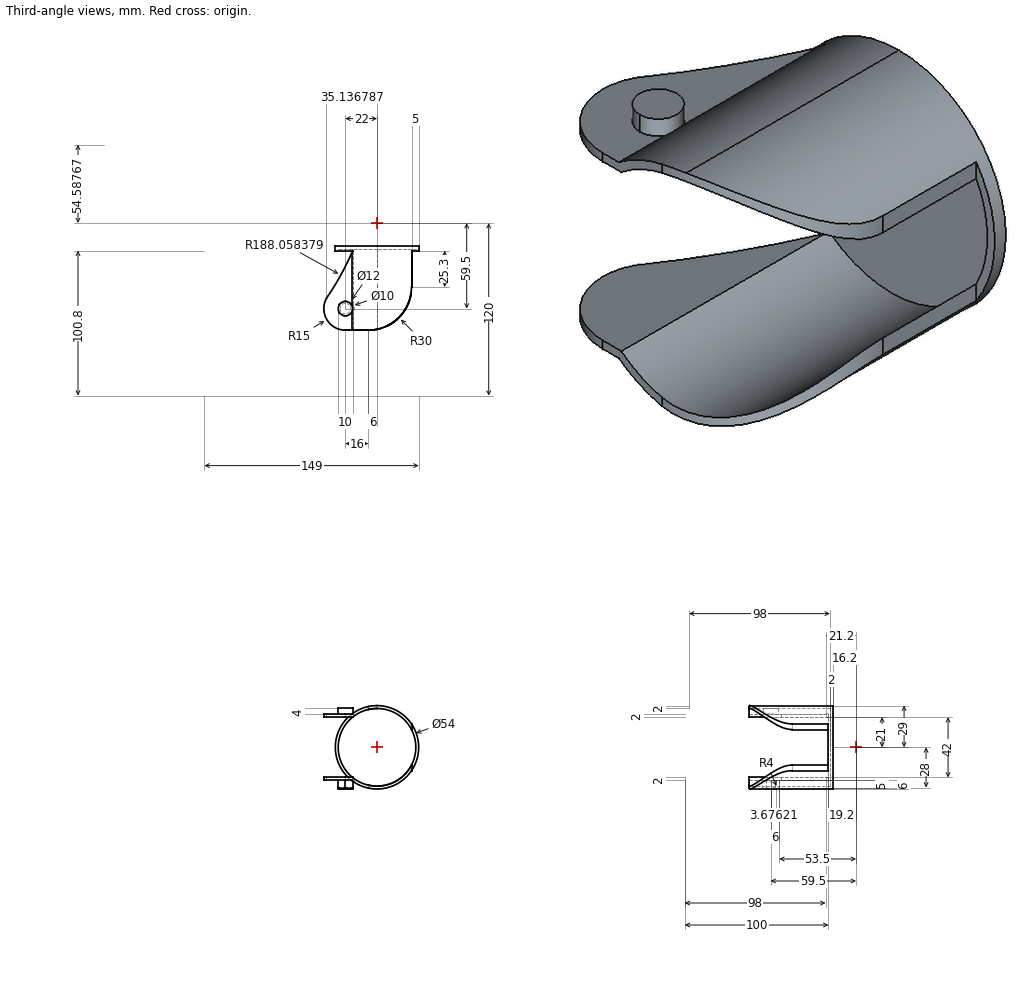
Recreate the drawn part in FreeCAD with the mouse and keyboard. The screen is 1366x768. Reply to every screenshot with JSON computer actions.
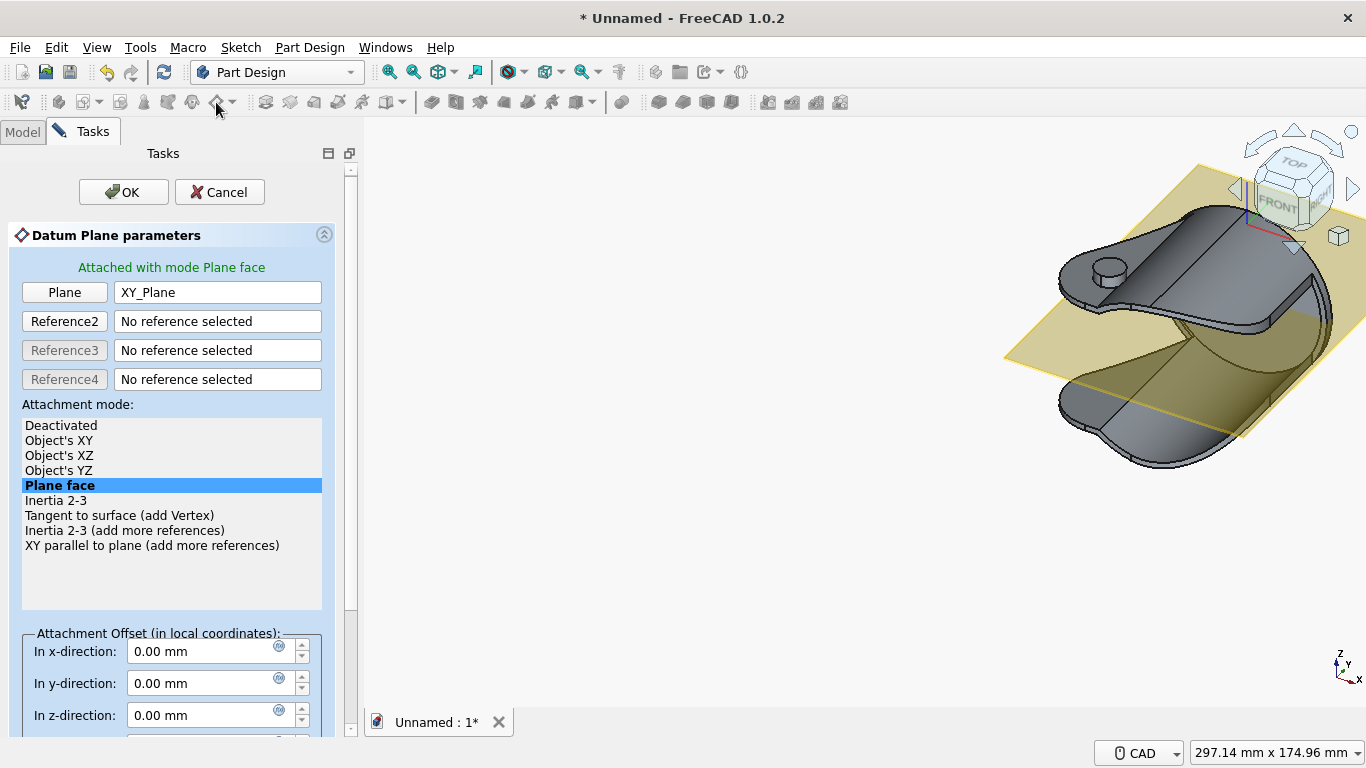
{"action": "triple_click", "coordinate": [210, 715]}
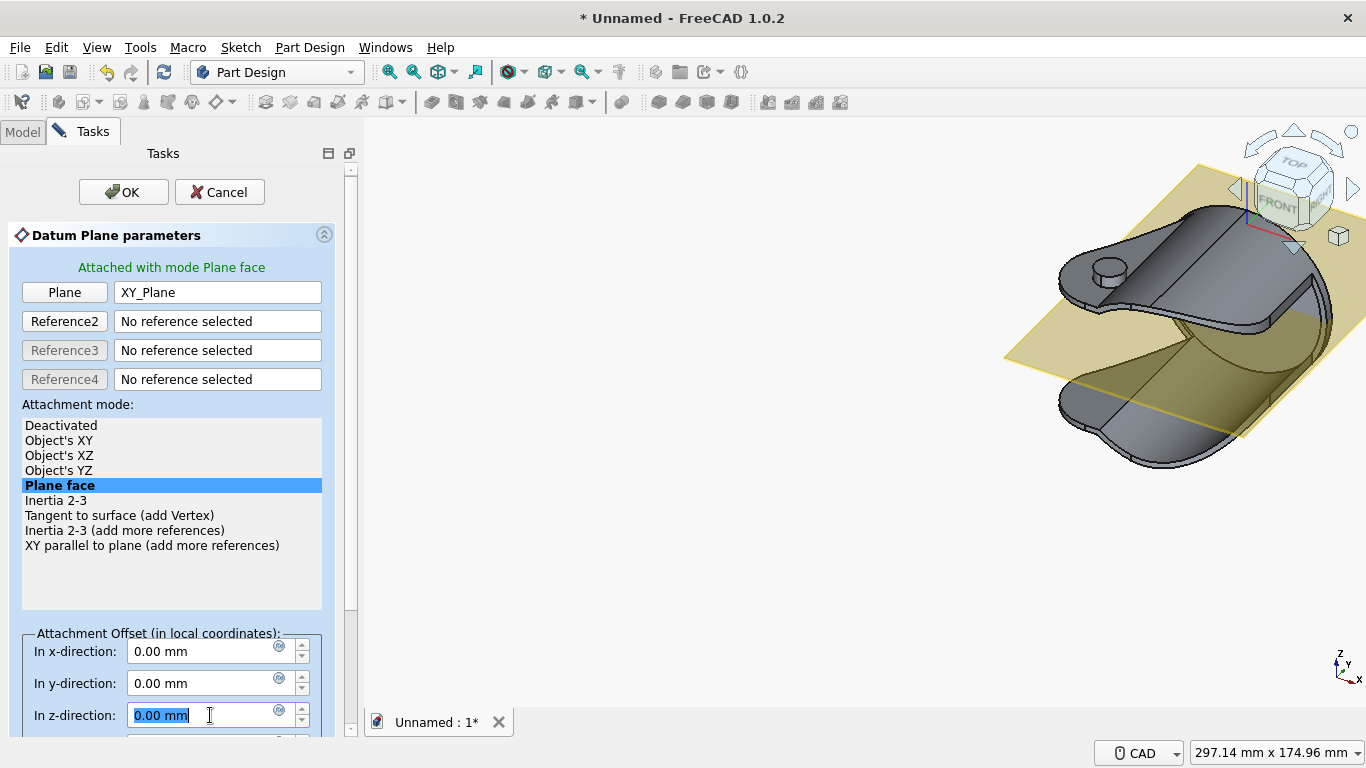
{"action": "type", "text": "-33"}
{"action": "key", "text": "Tab"}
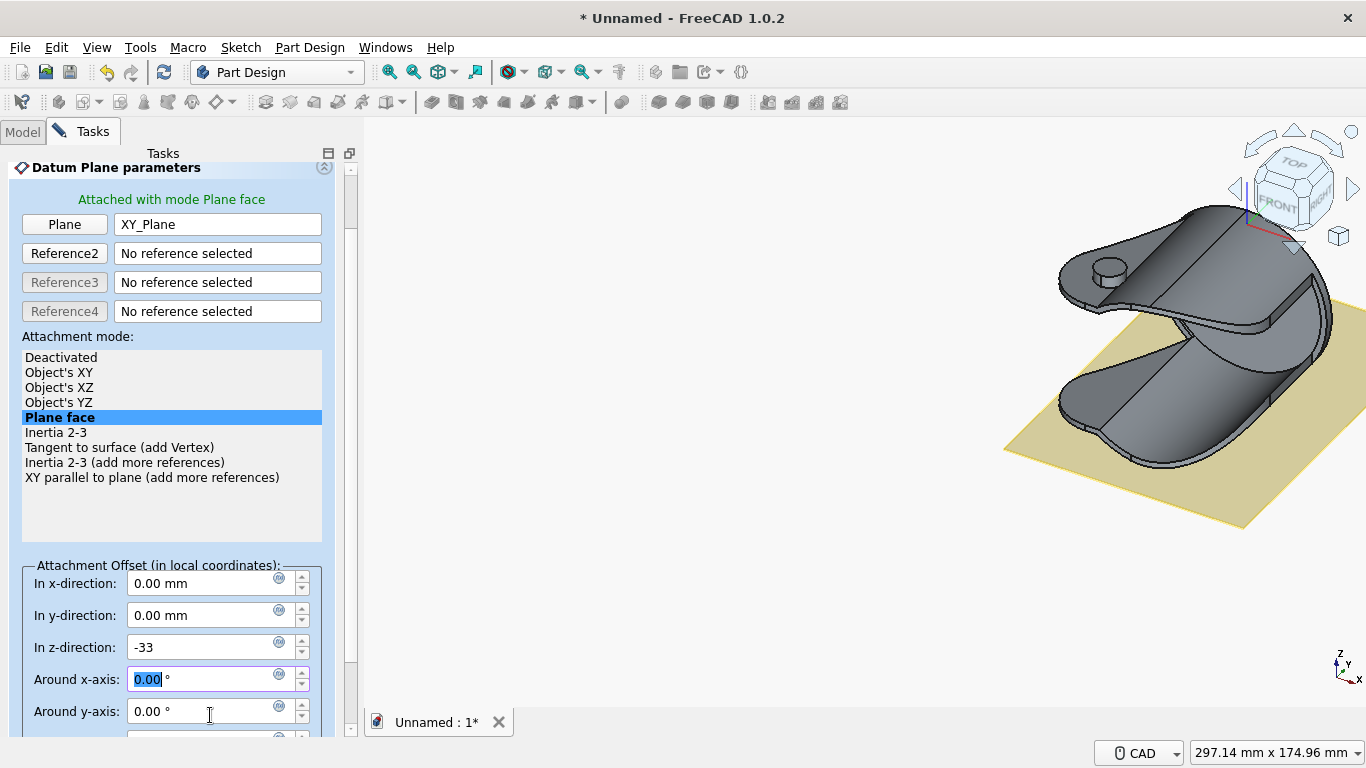
{"action": "scroll", "coordinate": [351, 450], "scroll_direction": "up", "scroll_amount": 2}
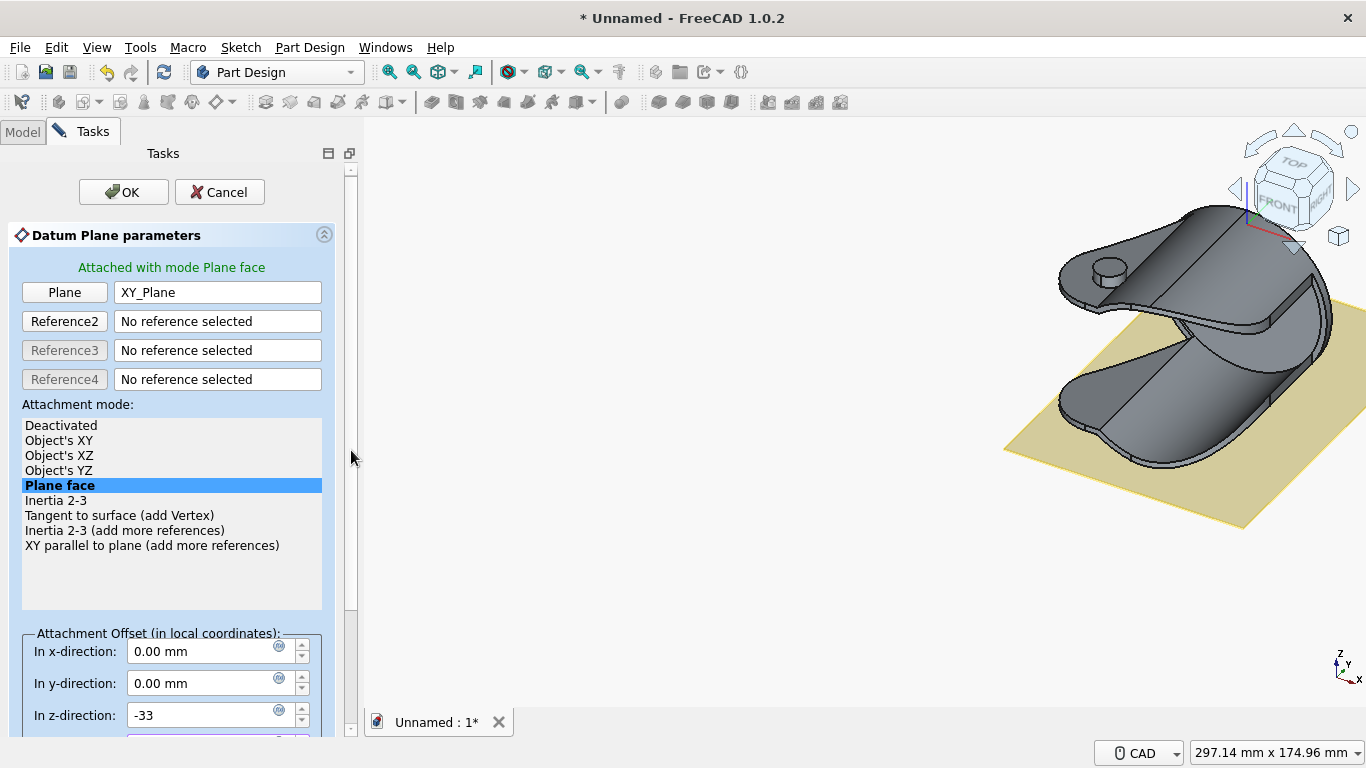
{"action": "left_click", "coordinate": [124, 192]}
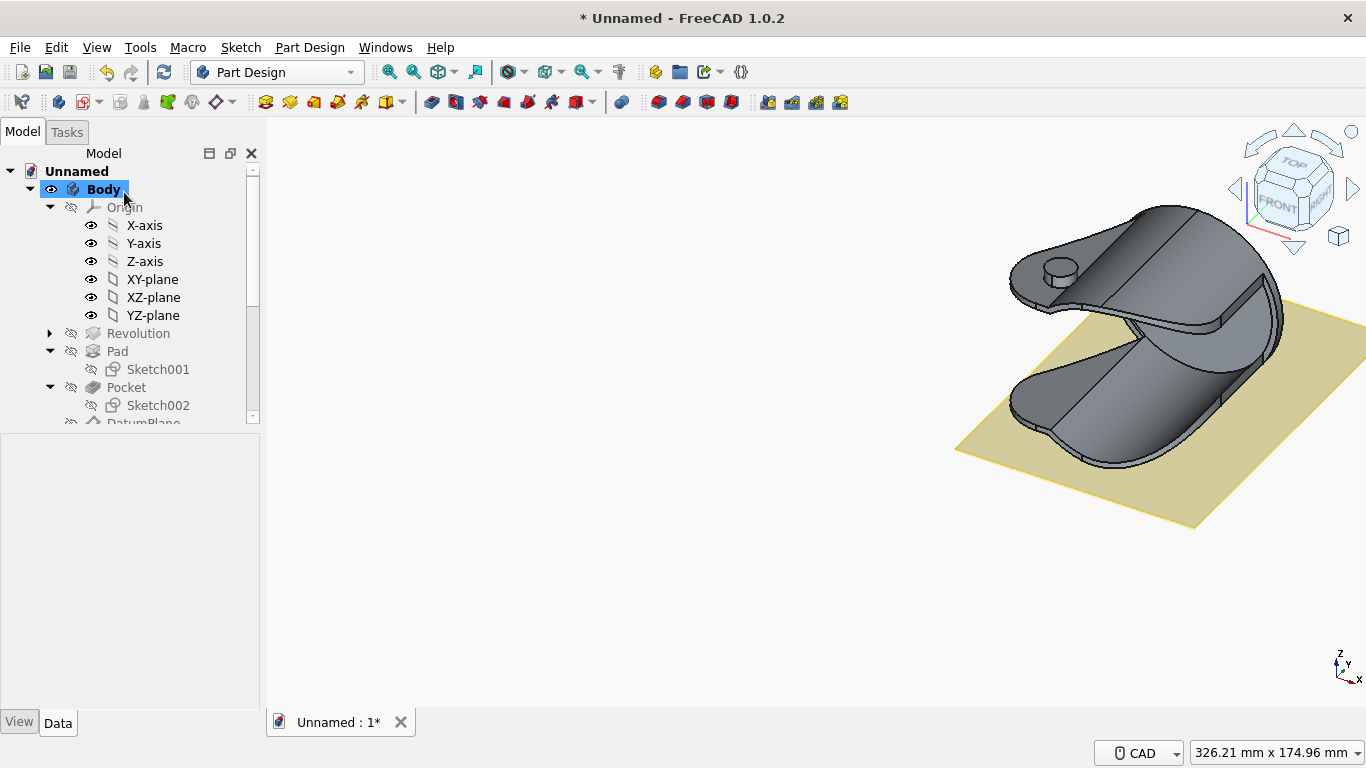
{"action": "scroll", "coordinate": [100, 293], "scroll_direction": "down", "scroll_amount": 3}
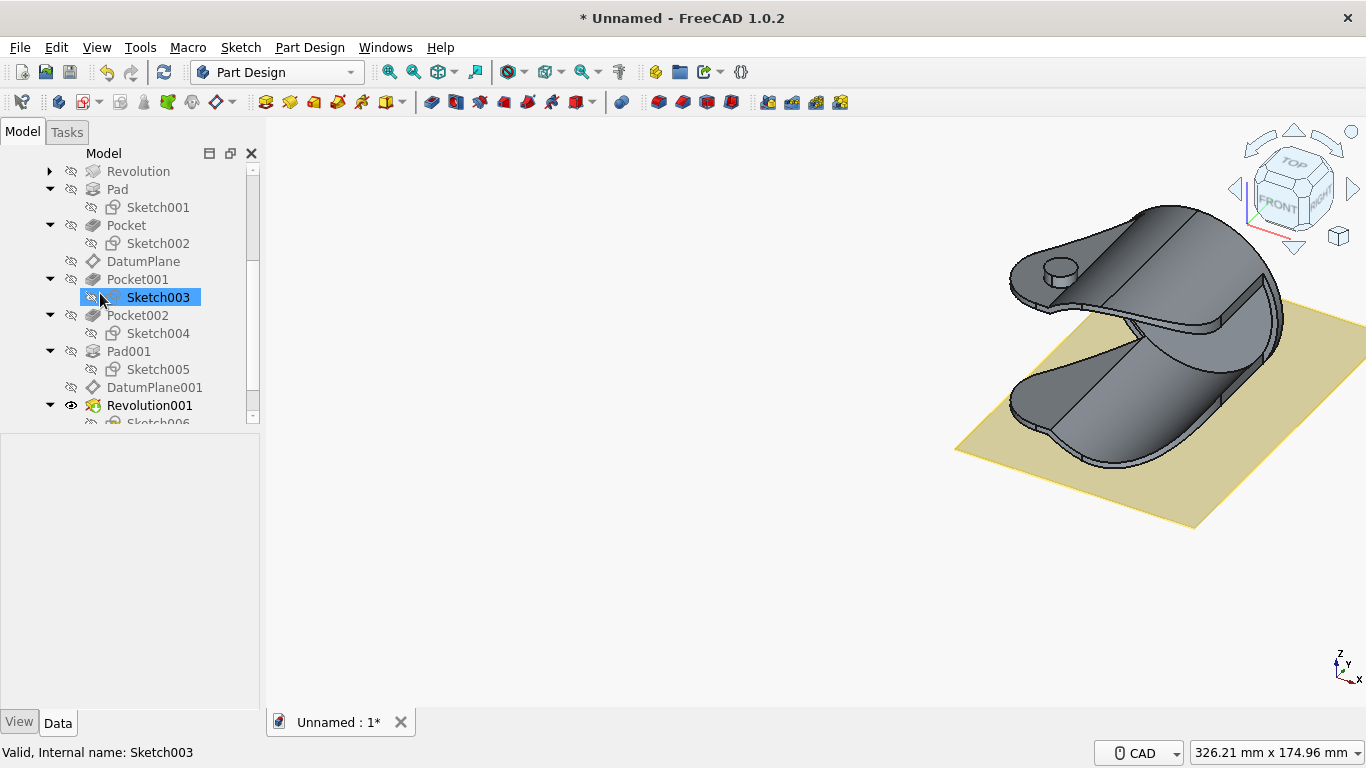
{"action": "scroll", "coordinate": [140, 293], "scroll_direction": "up", "scroll_amount": 15}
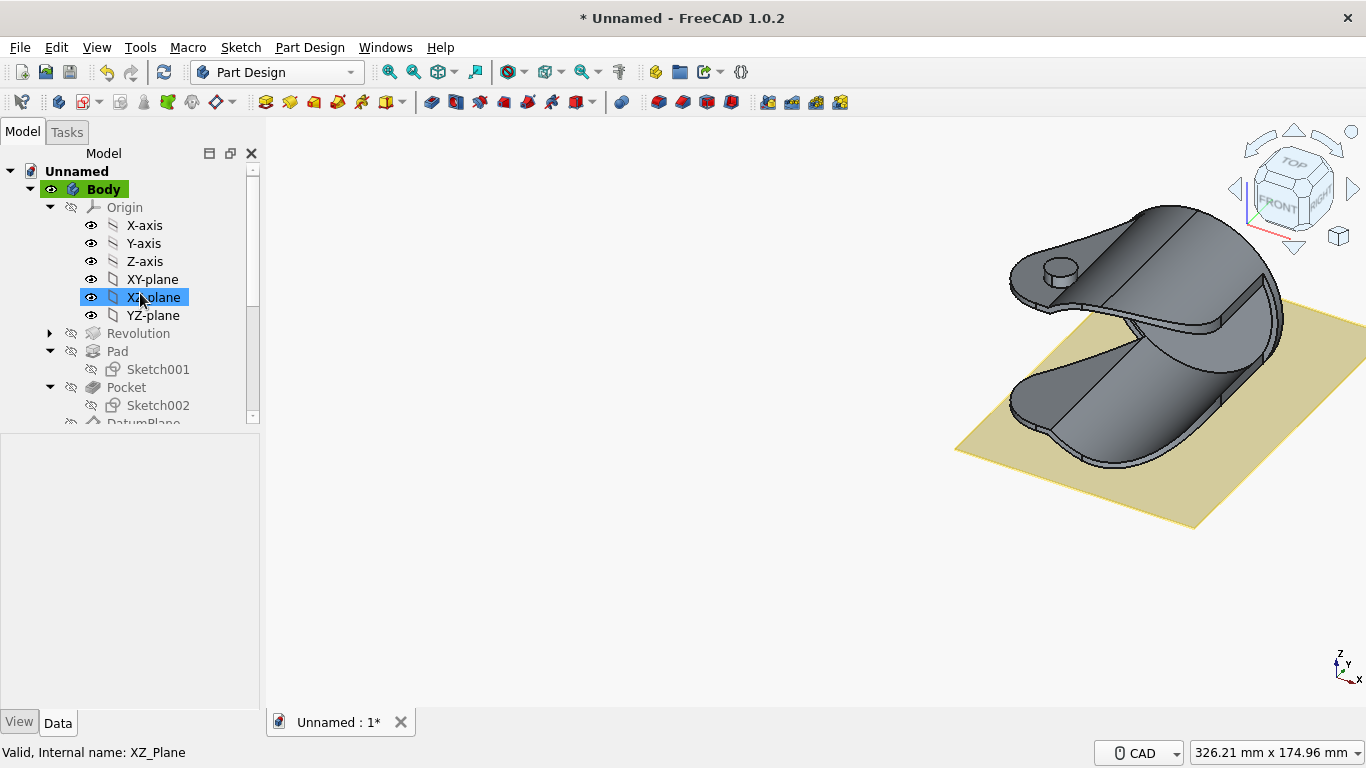
{"action": "scroll", "coordinate": [100, 293], "scroll_direction": "down", "scroll_amount": 6}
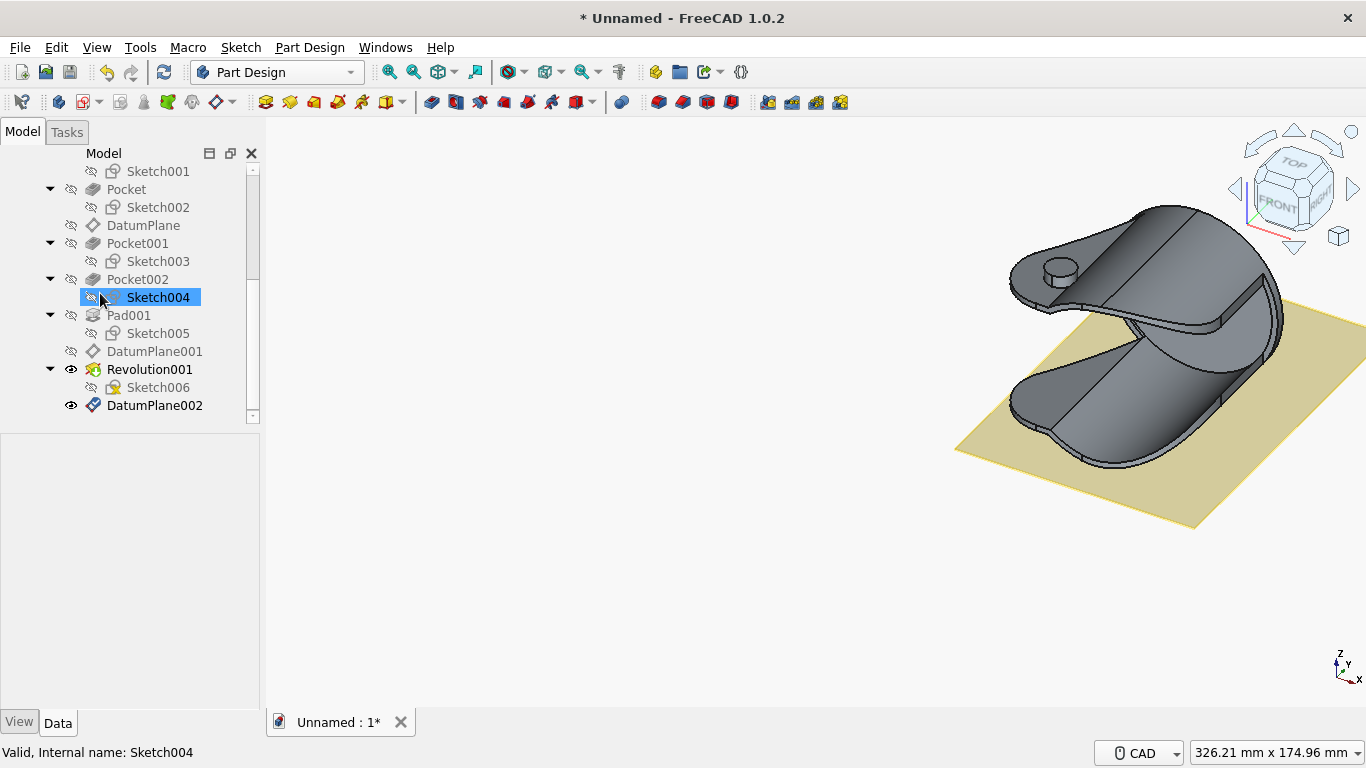
{"action": "left_click", "coordinate": [116, 405]}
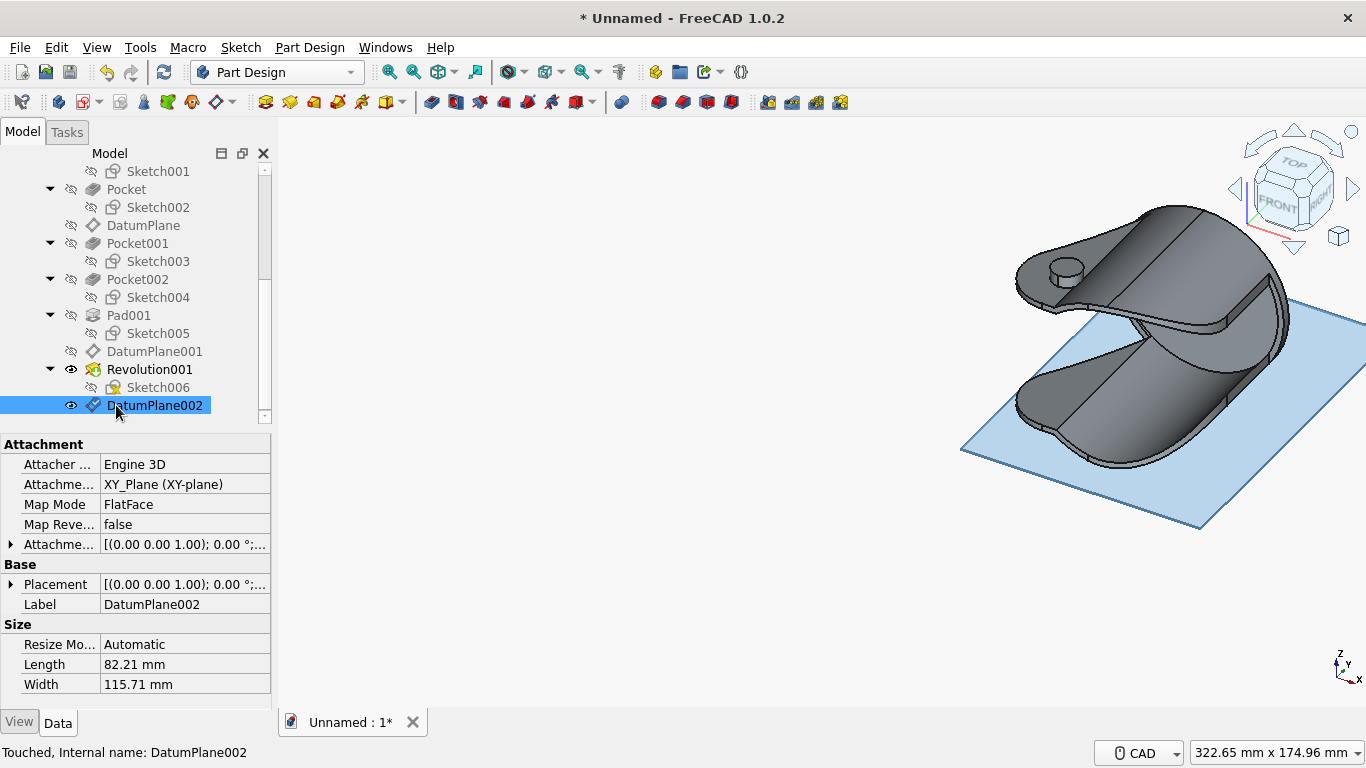
{"action": "left_click", "coordinate": [84, 102]}